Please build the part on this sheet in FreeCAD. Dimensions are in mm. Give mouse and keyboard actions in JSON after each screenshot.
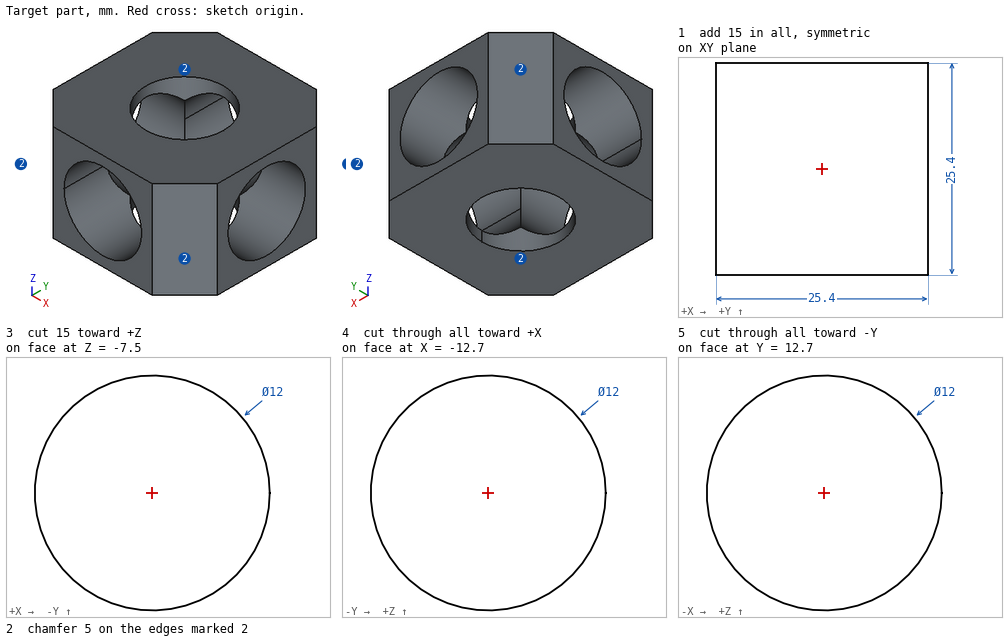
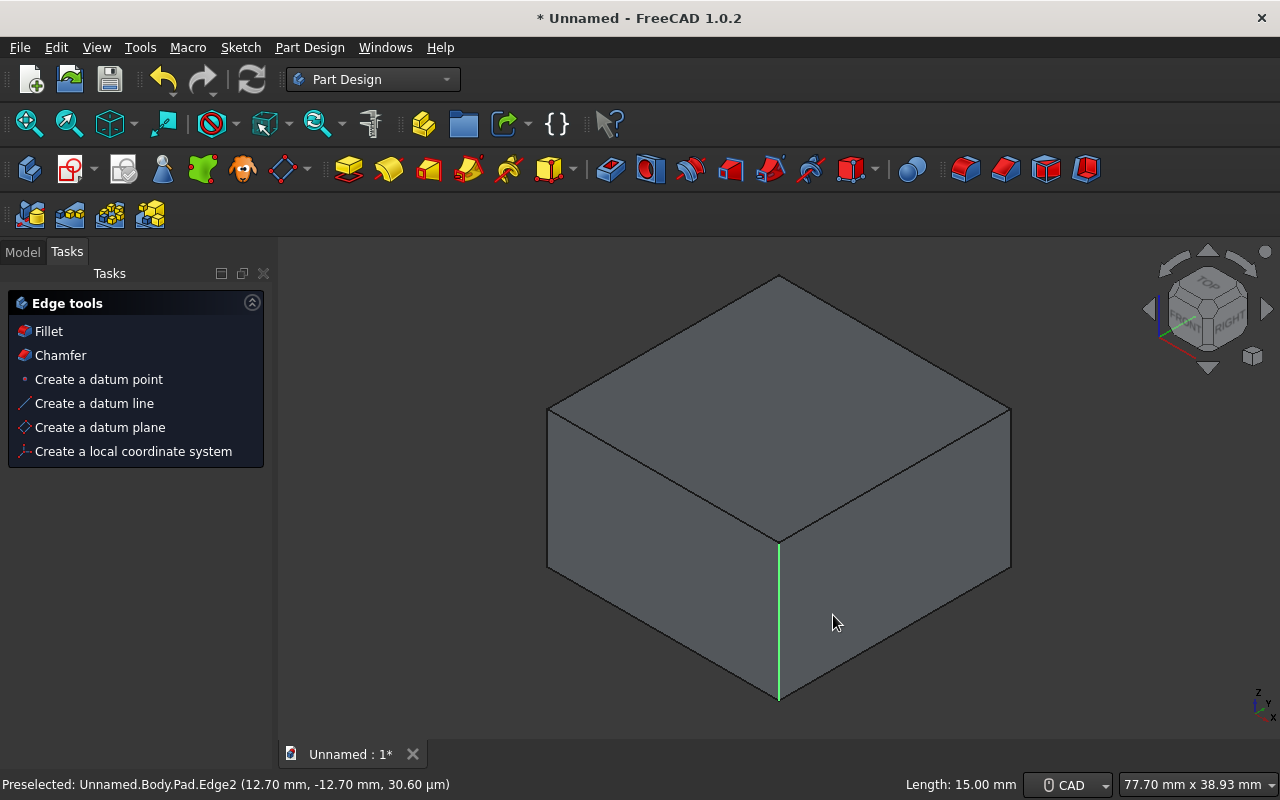
{"action": "key", "text": "2"}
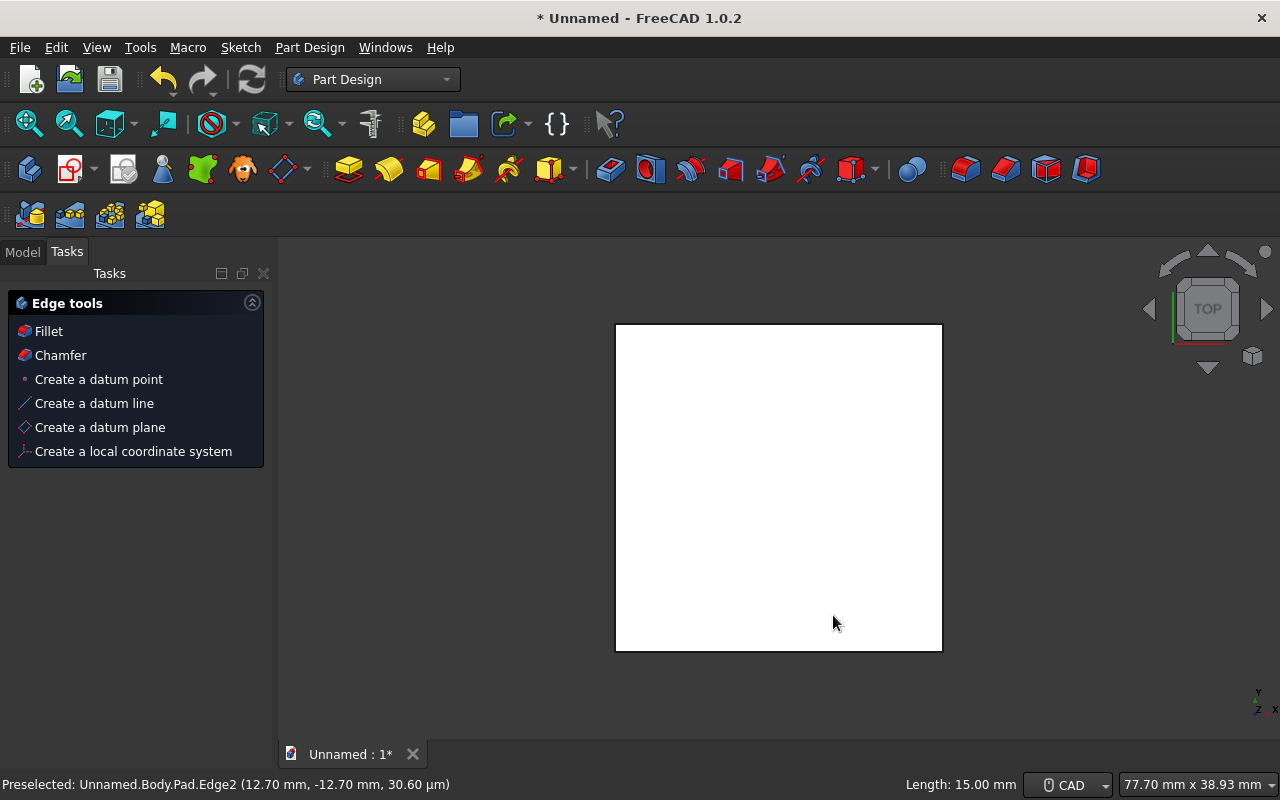
{"action": "key", "text": "1"}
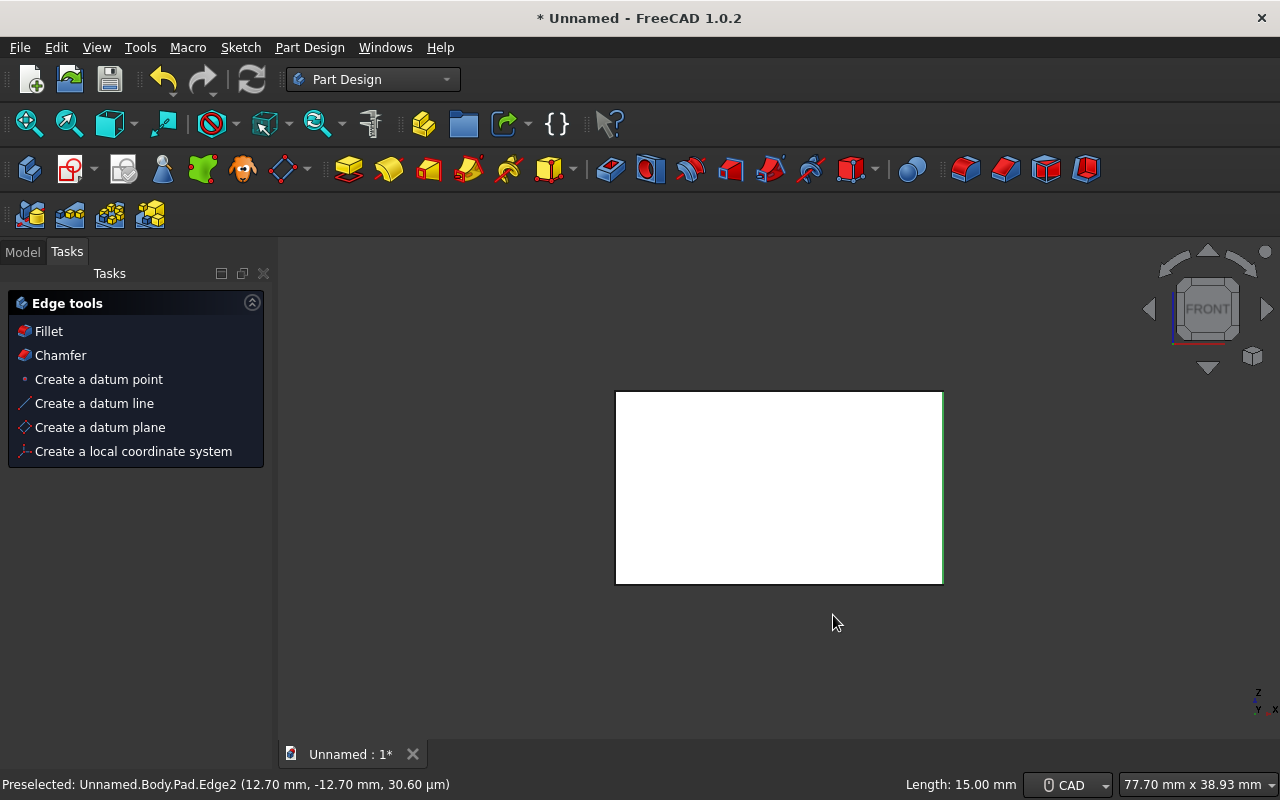
{"action": "key", "text": "v f"}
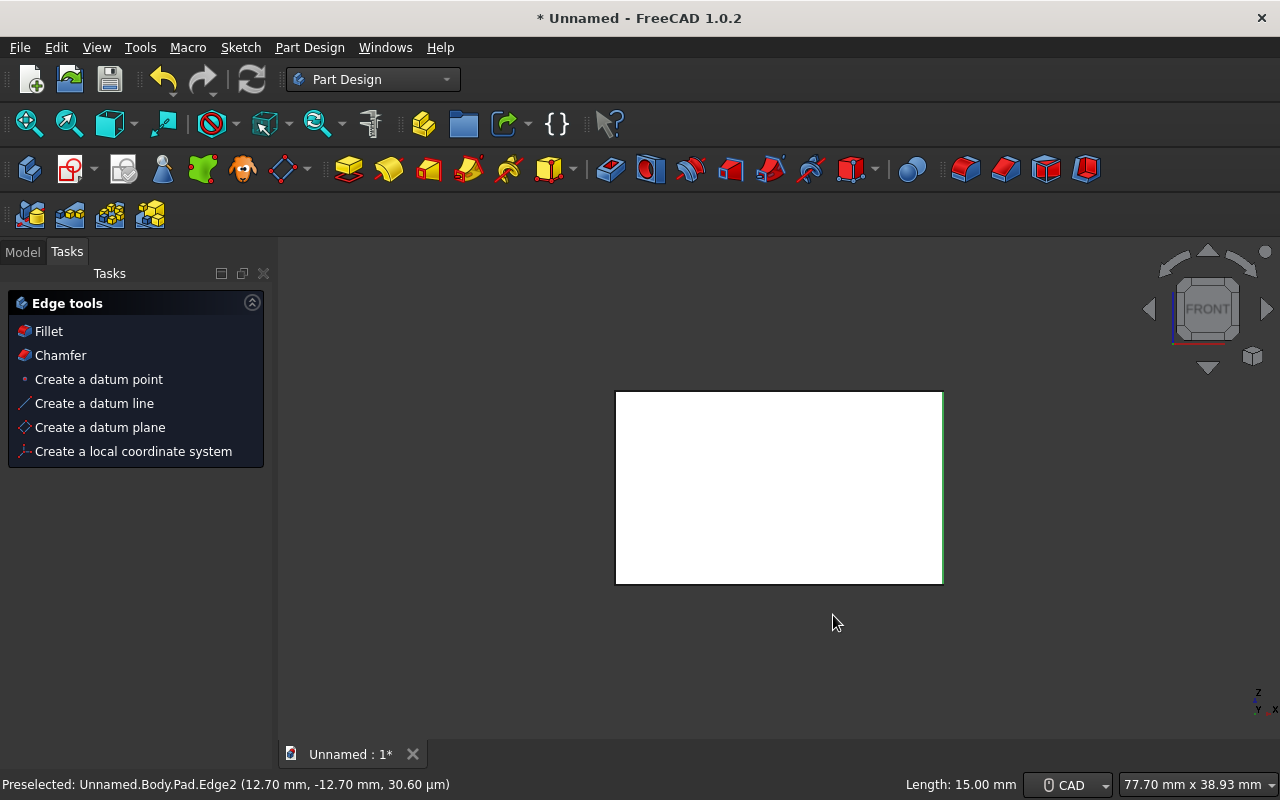
{"action": "left_click", "coordinate": [615, 487], "text": "ctrl"}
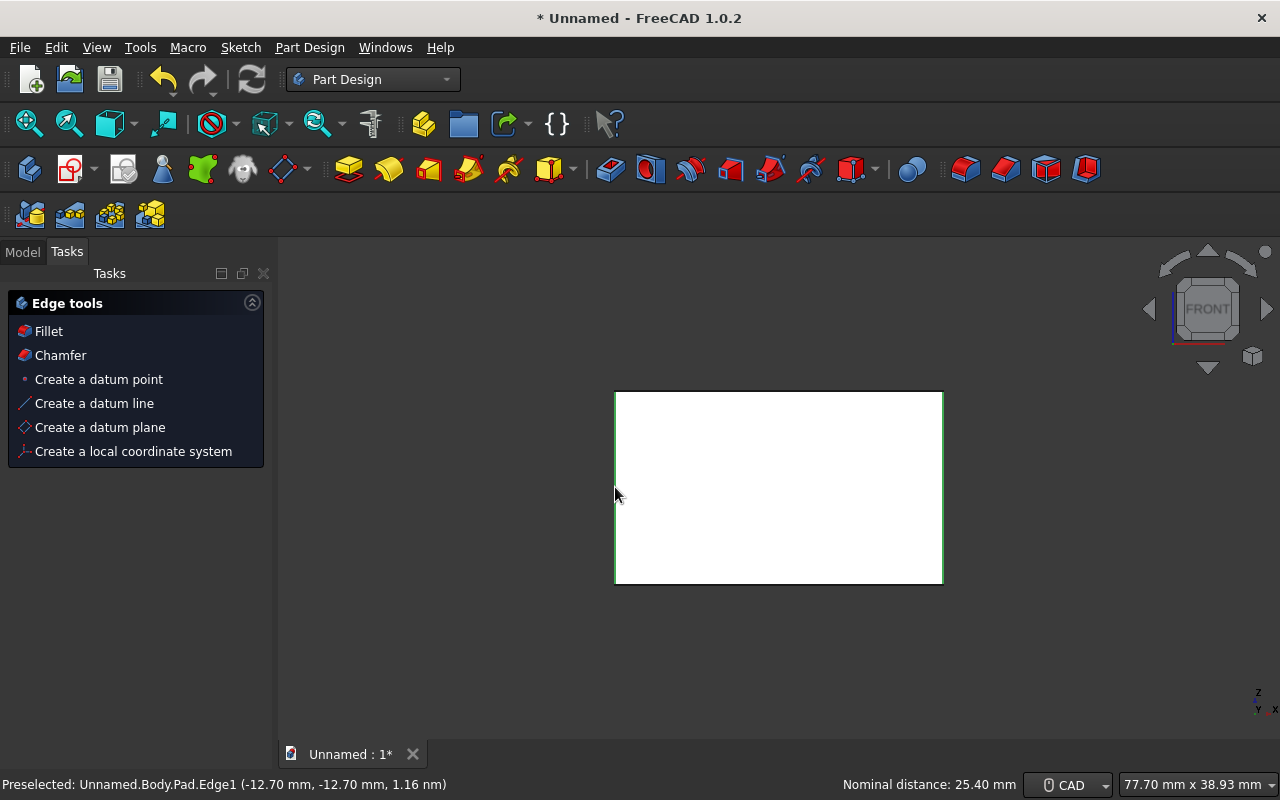
{"action": "key", "text": "3"}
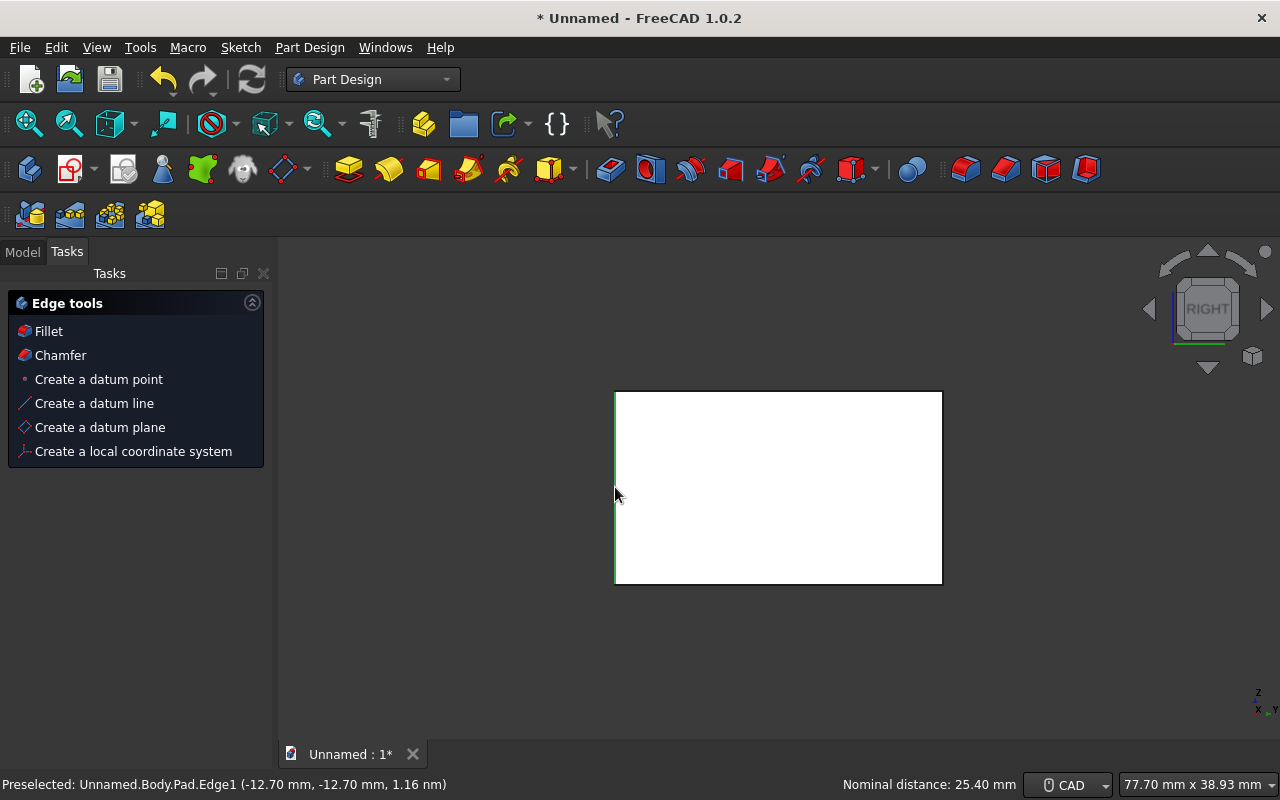
{"action": "key", "text": "v f"}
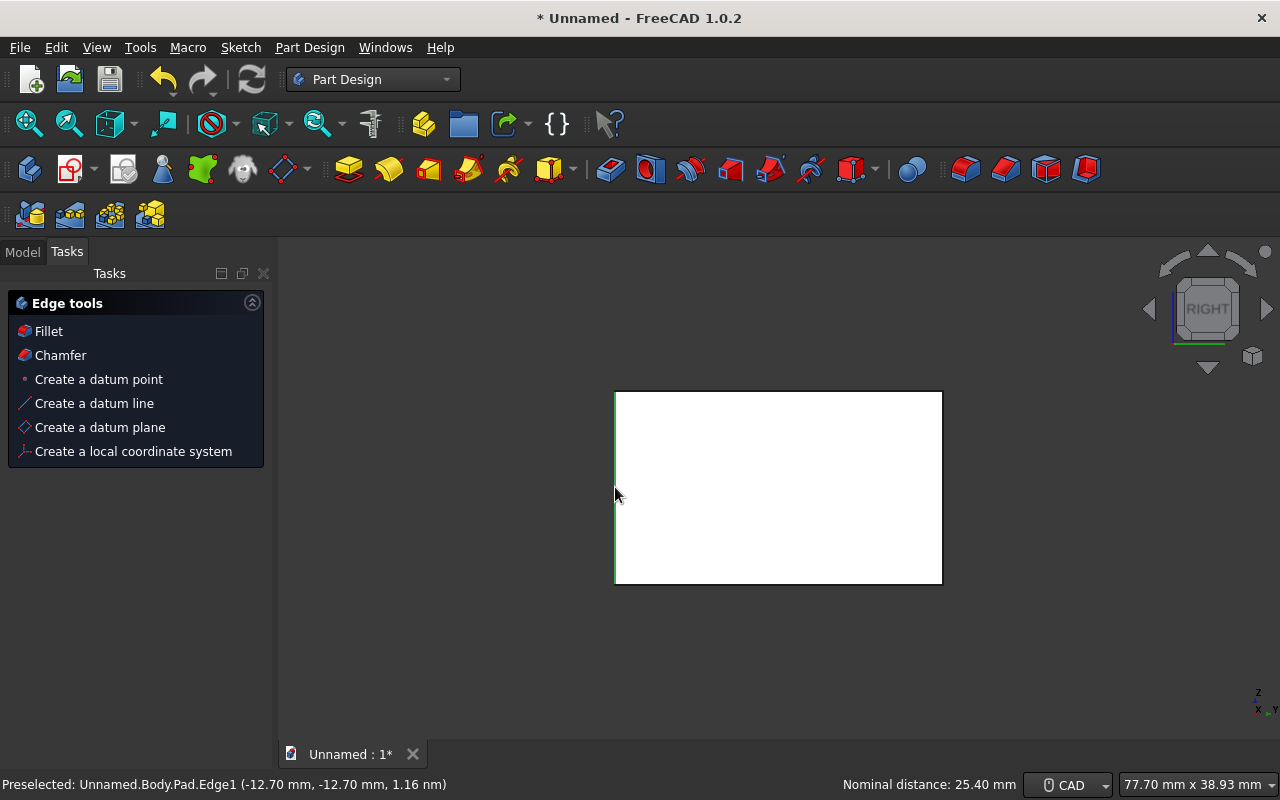
{"action": "left_click", "coordinate": [943, 487], "text": "ctrl"}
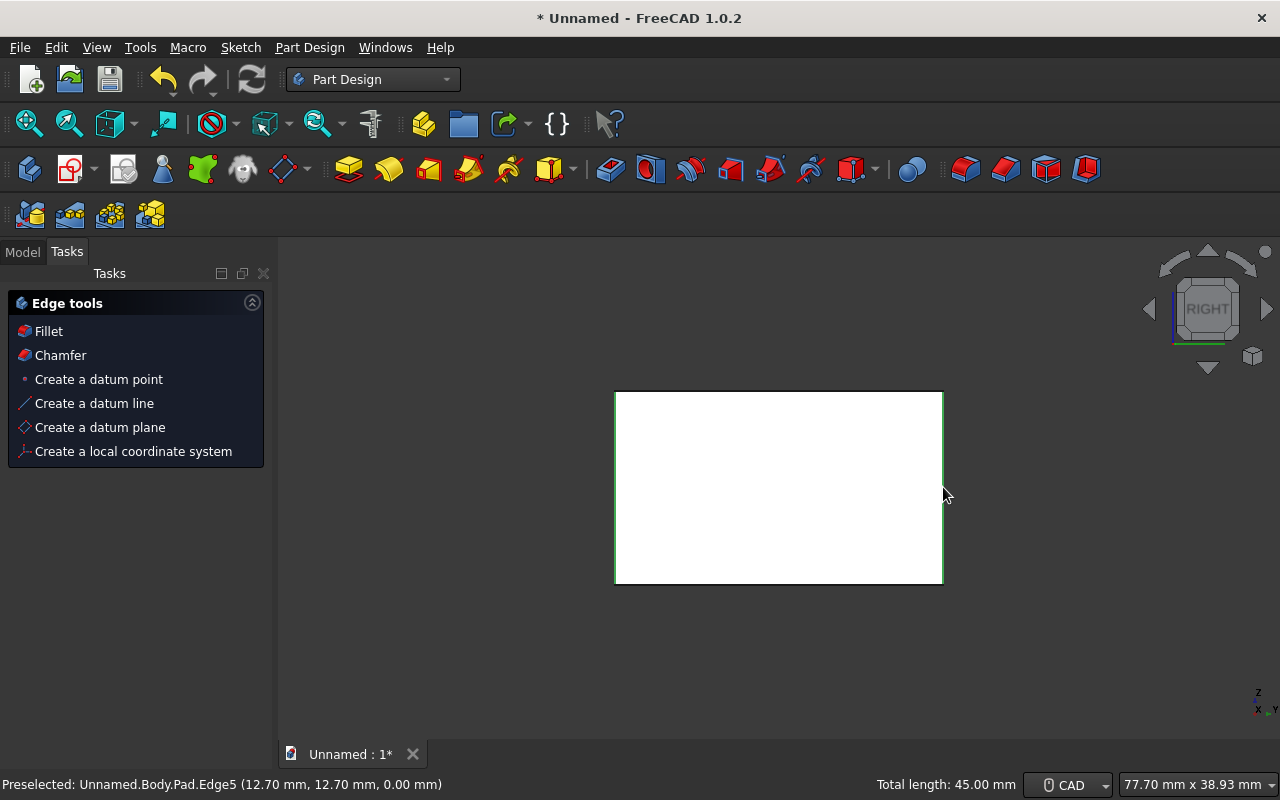
{"action": "key", "text": "5"}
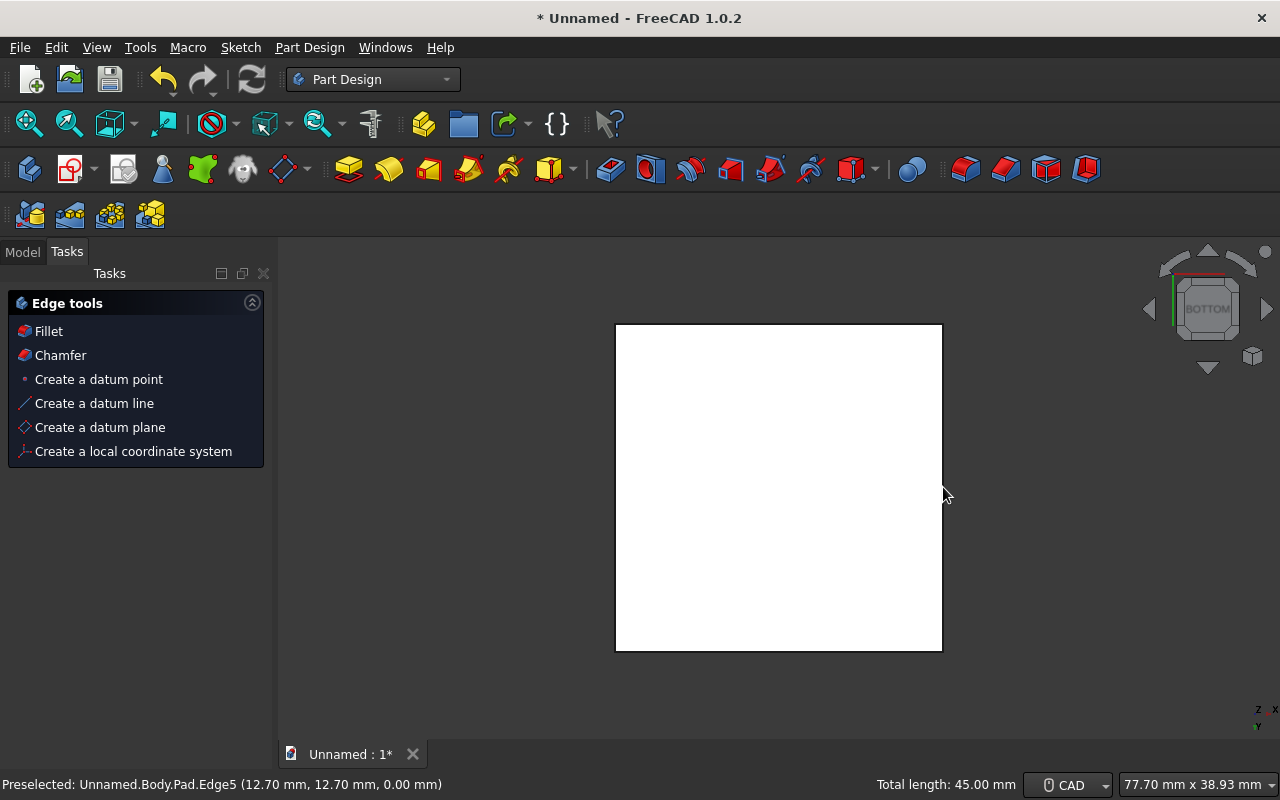
{"action": "key", "text": "4"}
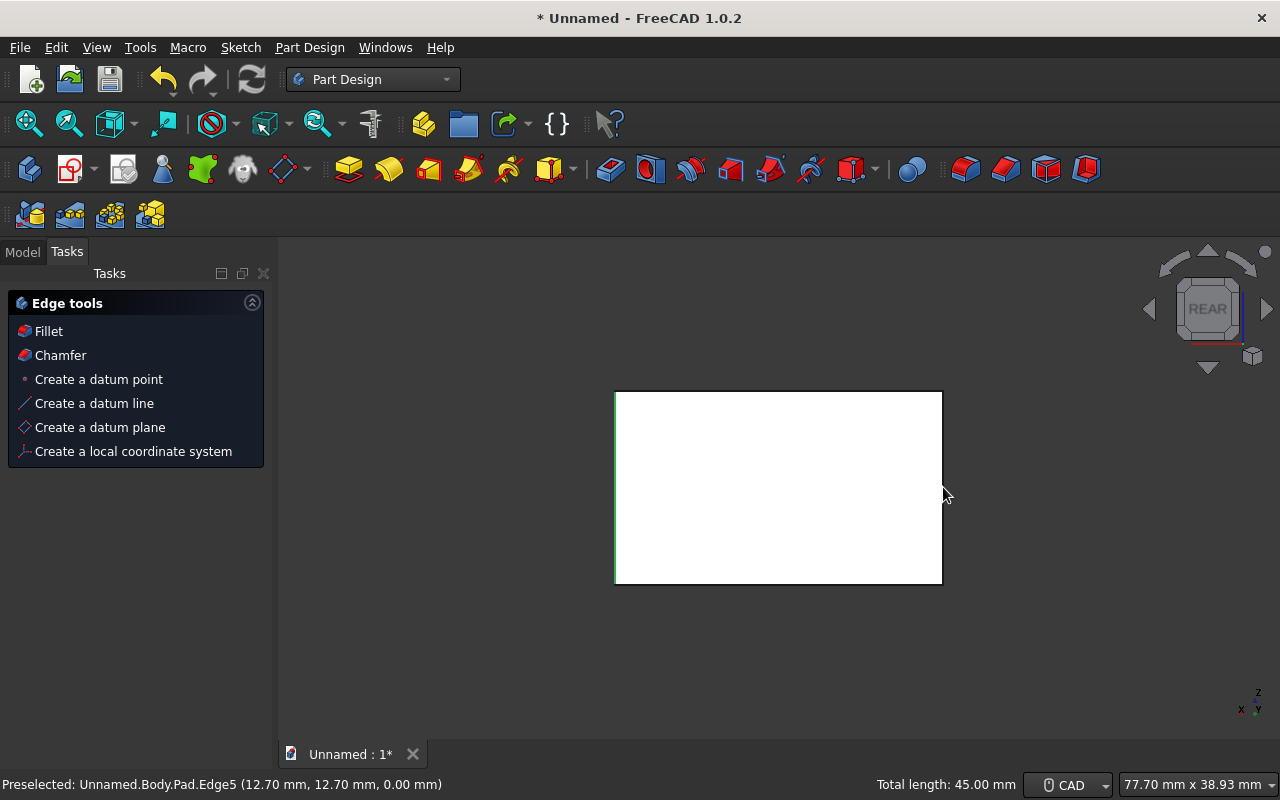
{"action": "key", "text": "v f"}